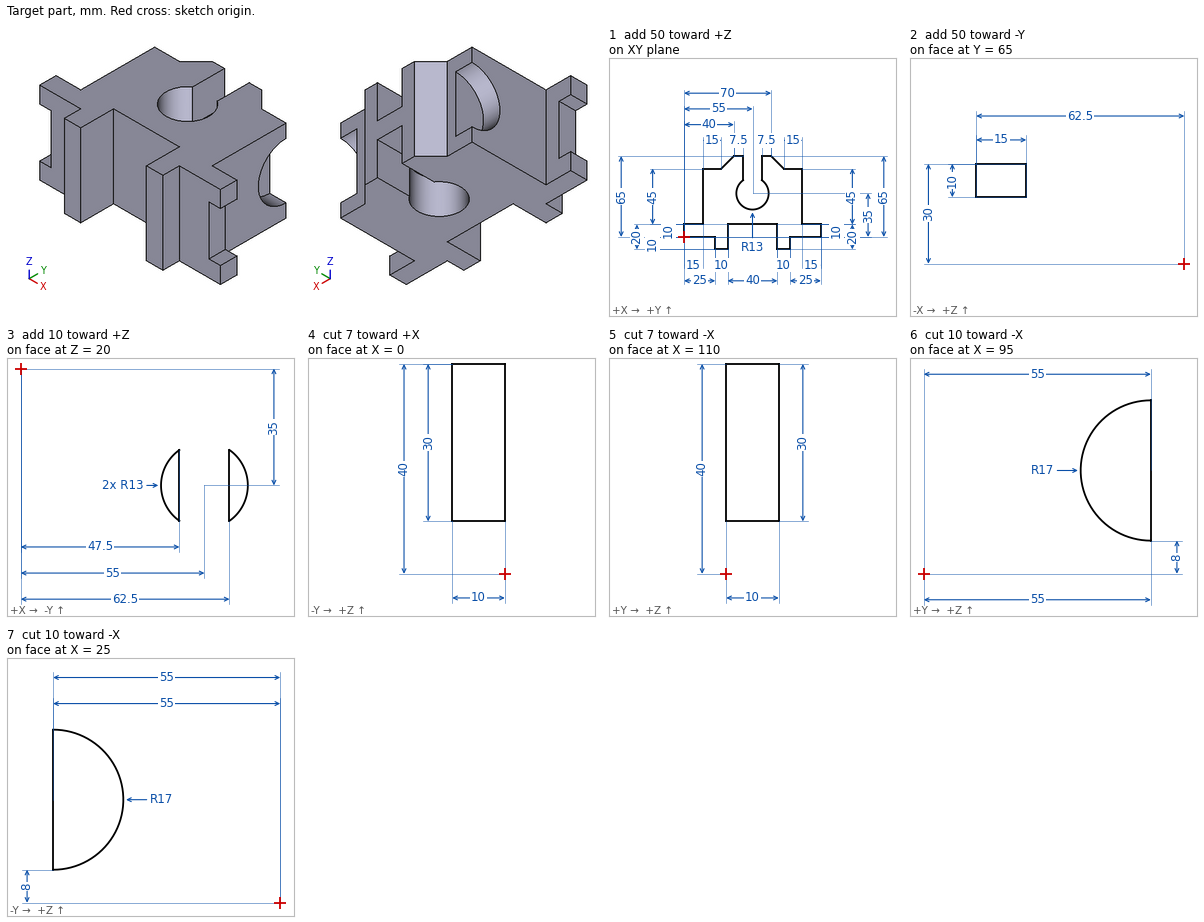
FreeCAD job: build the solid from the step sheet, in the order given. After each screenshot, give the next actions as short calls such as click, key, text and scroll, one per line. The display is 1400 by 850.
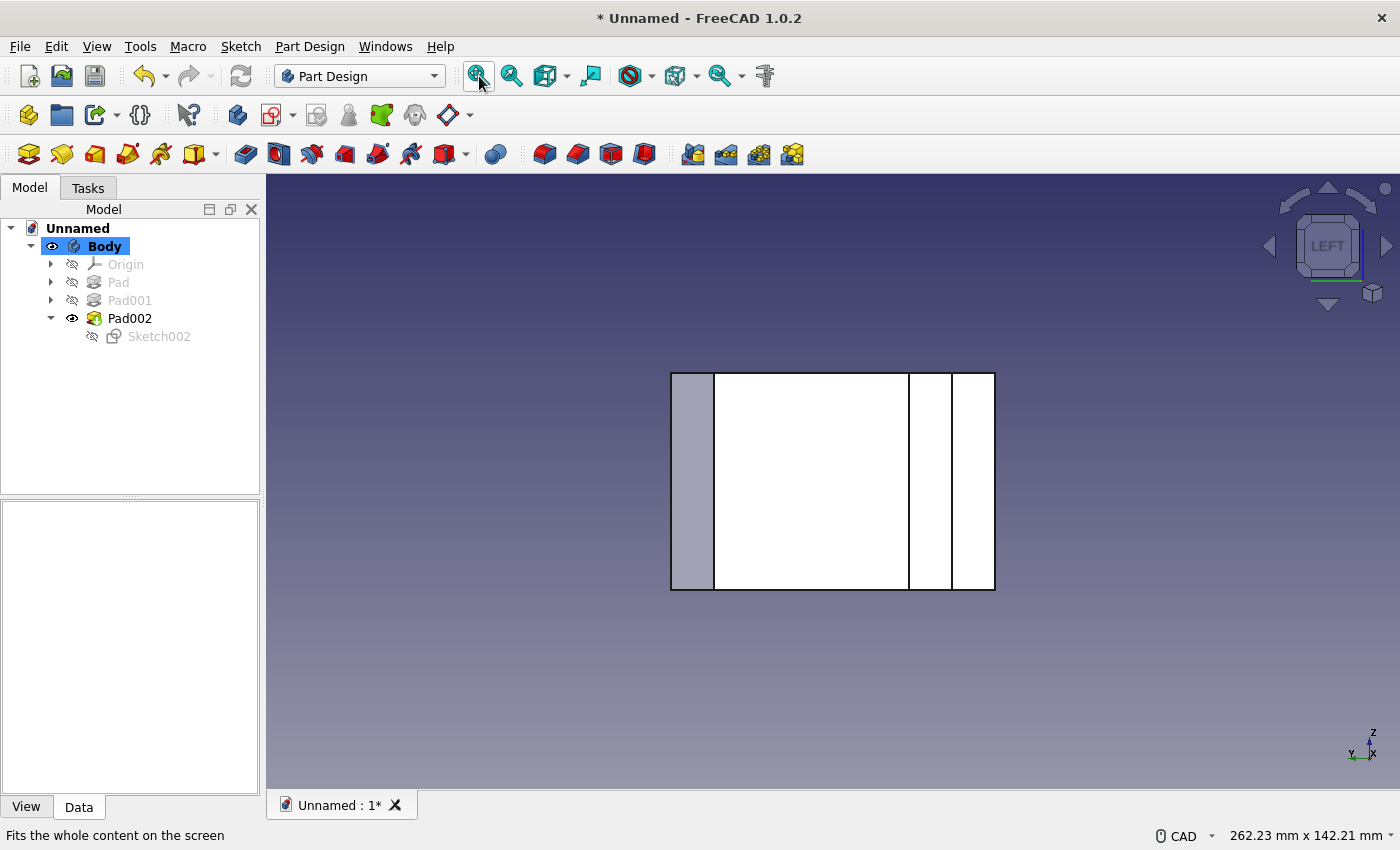
click(930, 419)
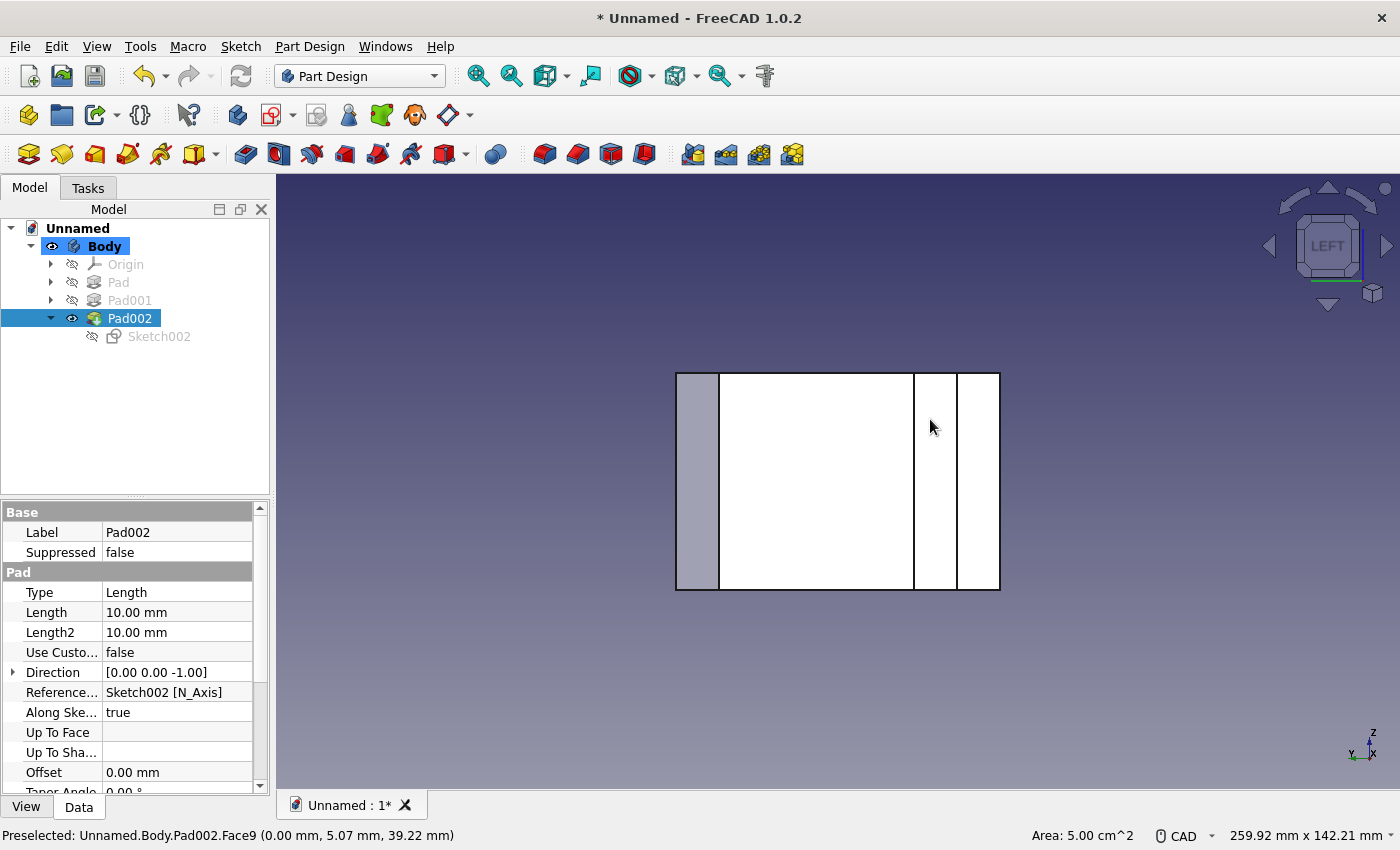
click(270, 116)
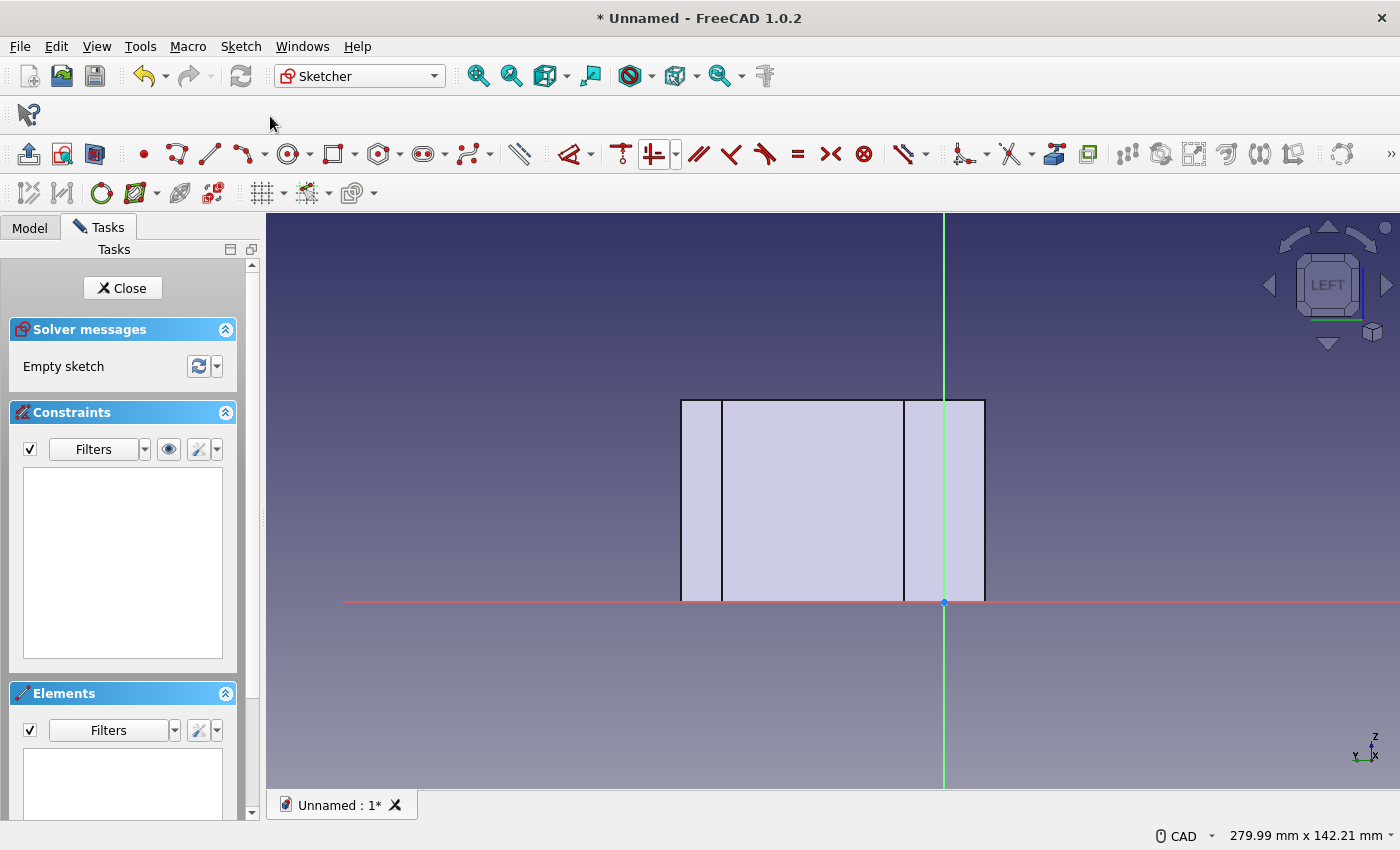
scroll(1054, 538, up, 4)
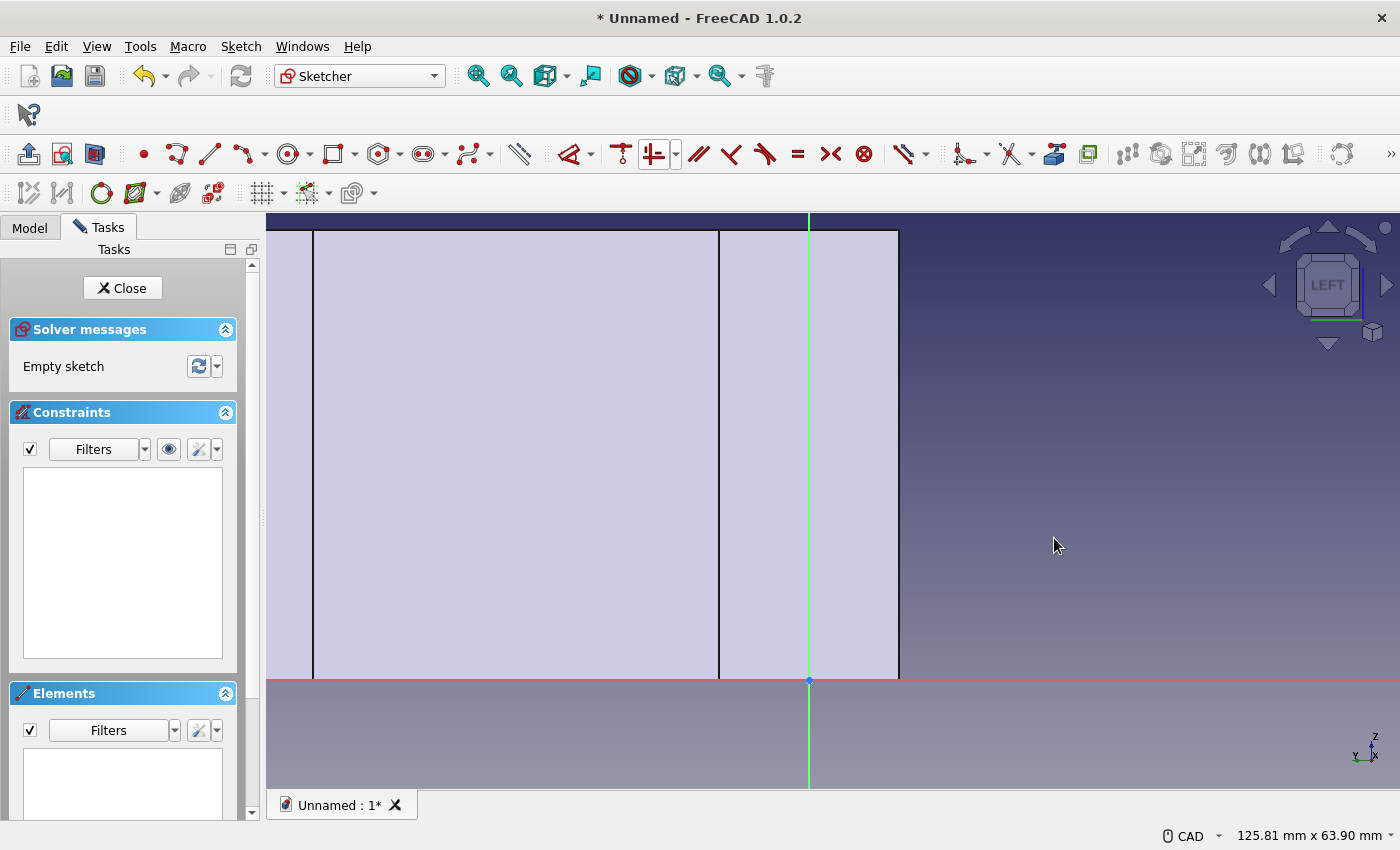
click(332, 154)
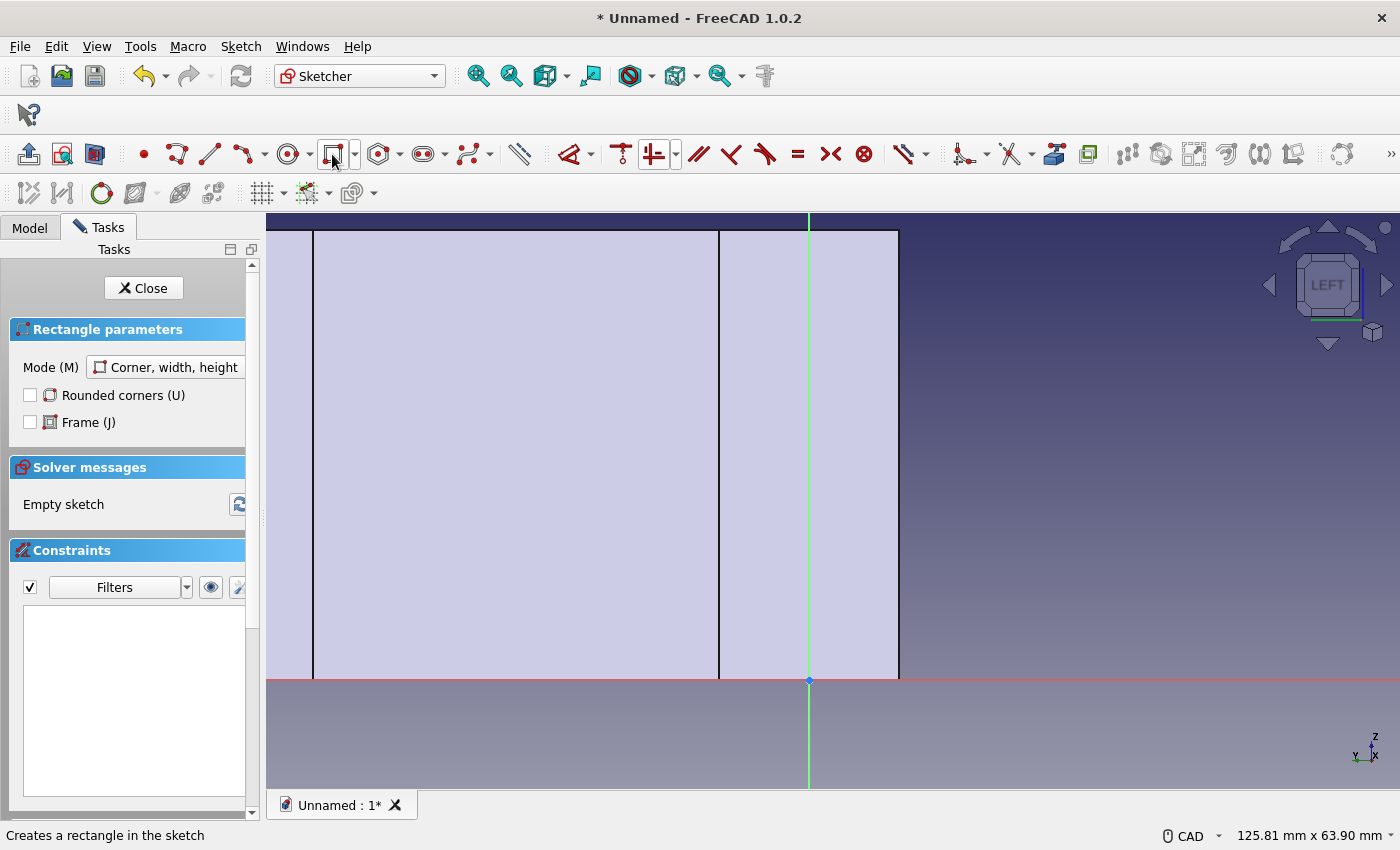
click(719, 320)
click(809, 590)
key(Escape)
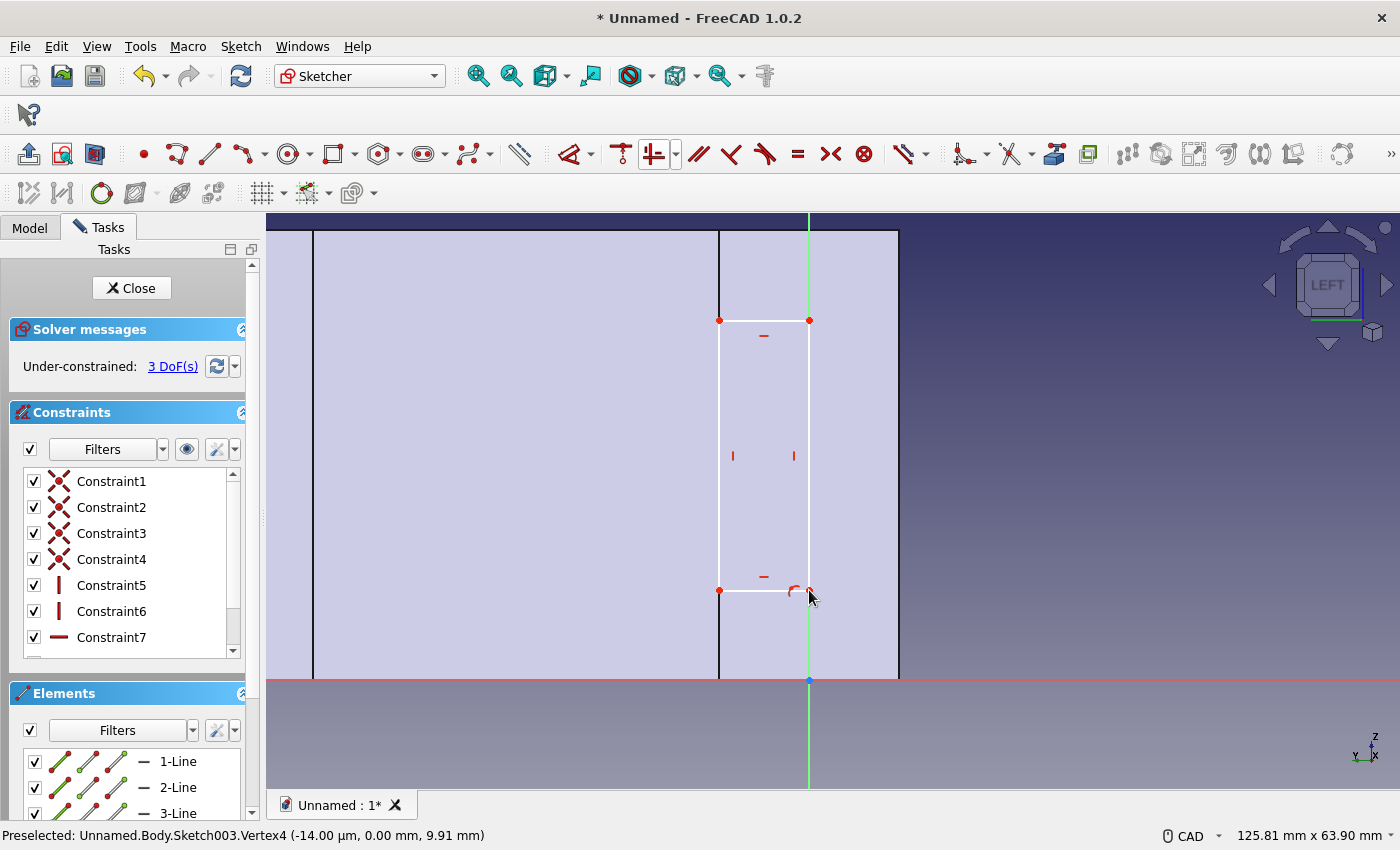
click(568, 154)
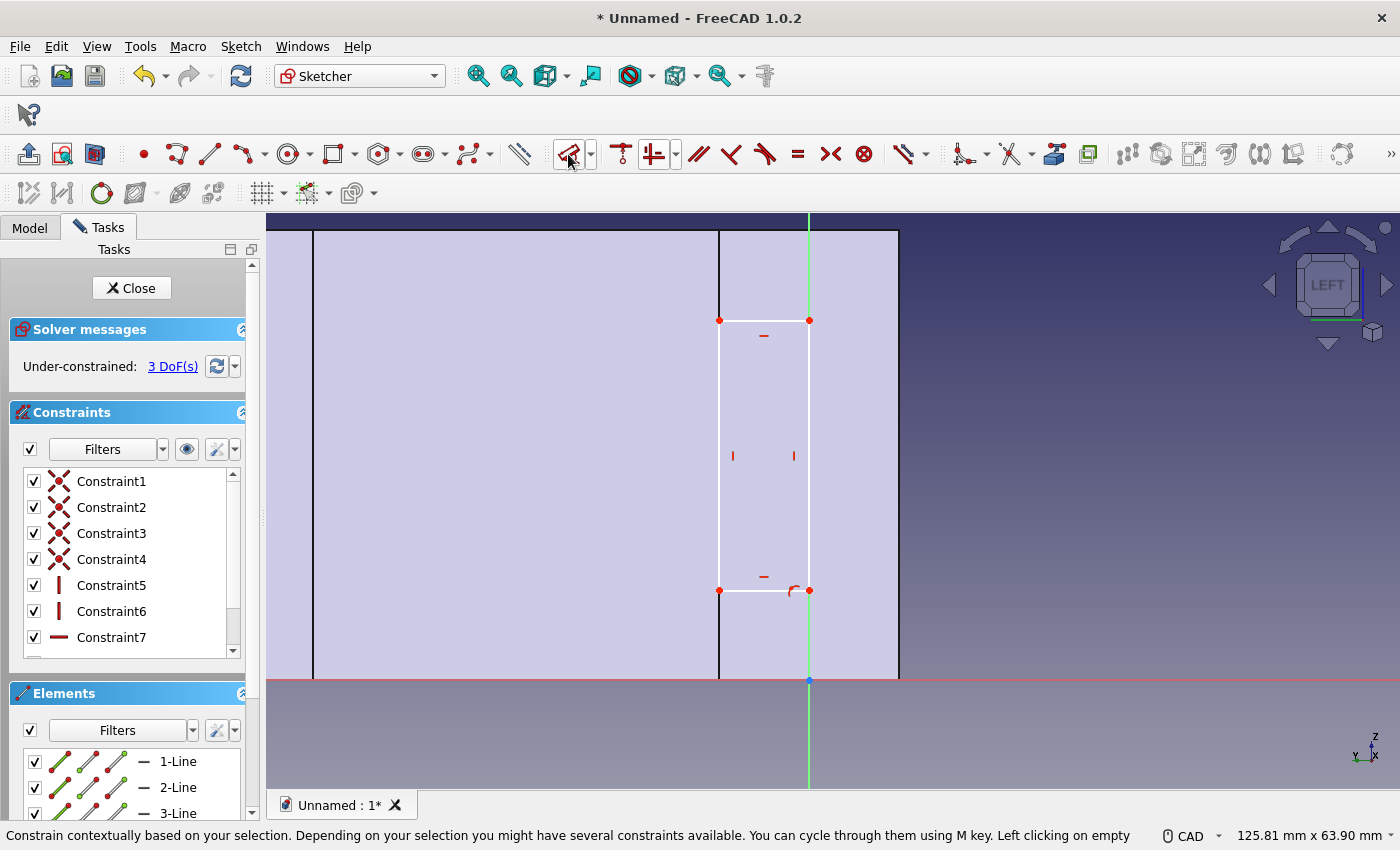
click(719, 402)
click(685, 456)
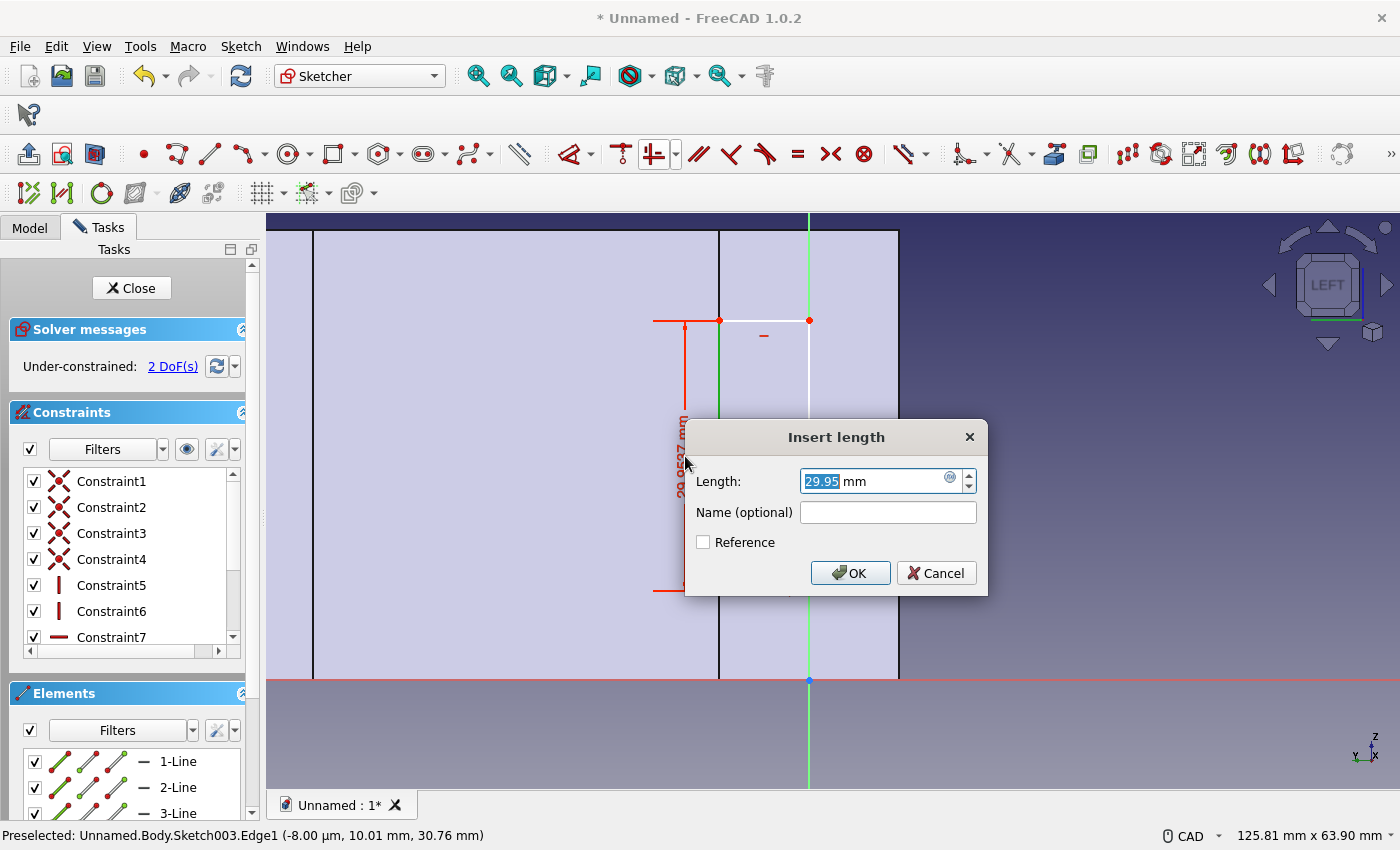
text(30)
key(Return)